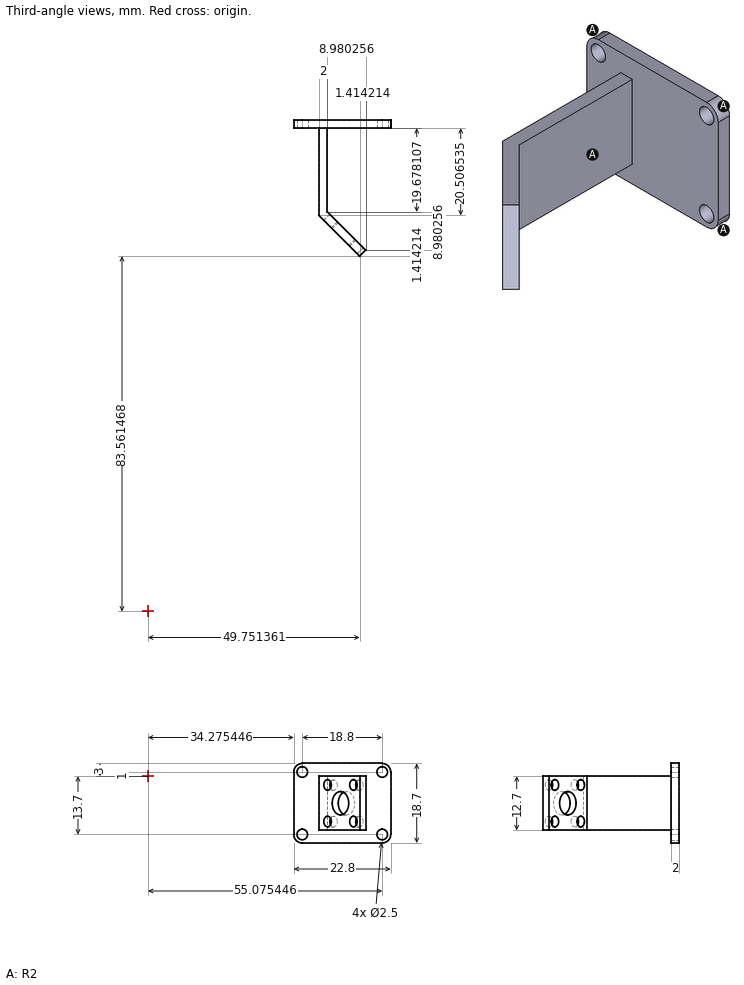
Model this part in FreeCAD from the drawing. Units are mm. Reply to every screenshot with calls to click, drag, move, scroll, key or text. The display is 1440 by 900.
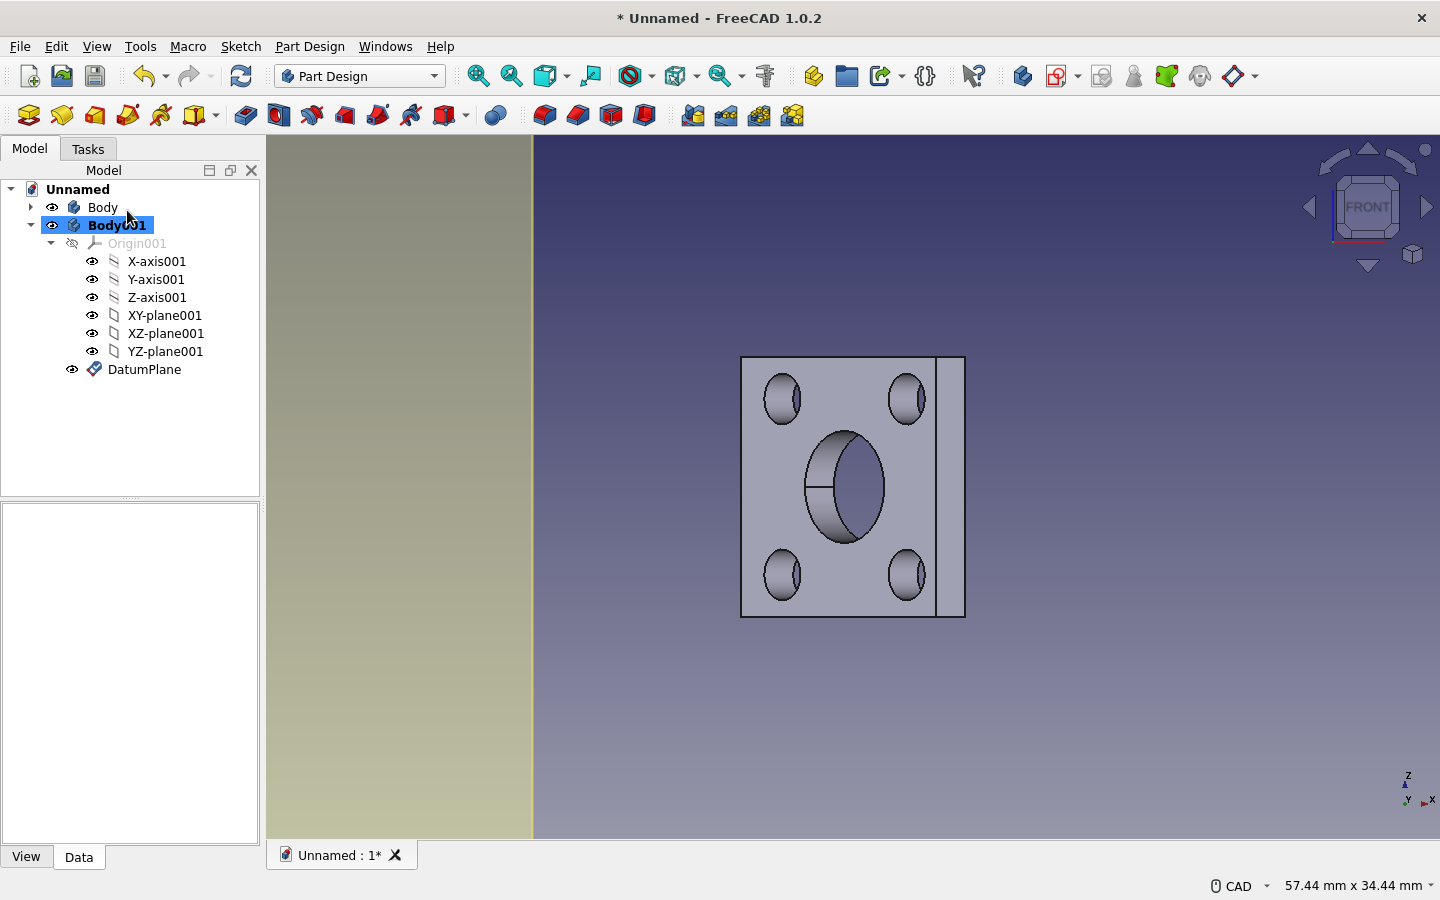
click(117, 369)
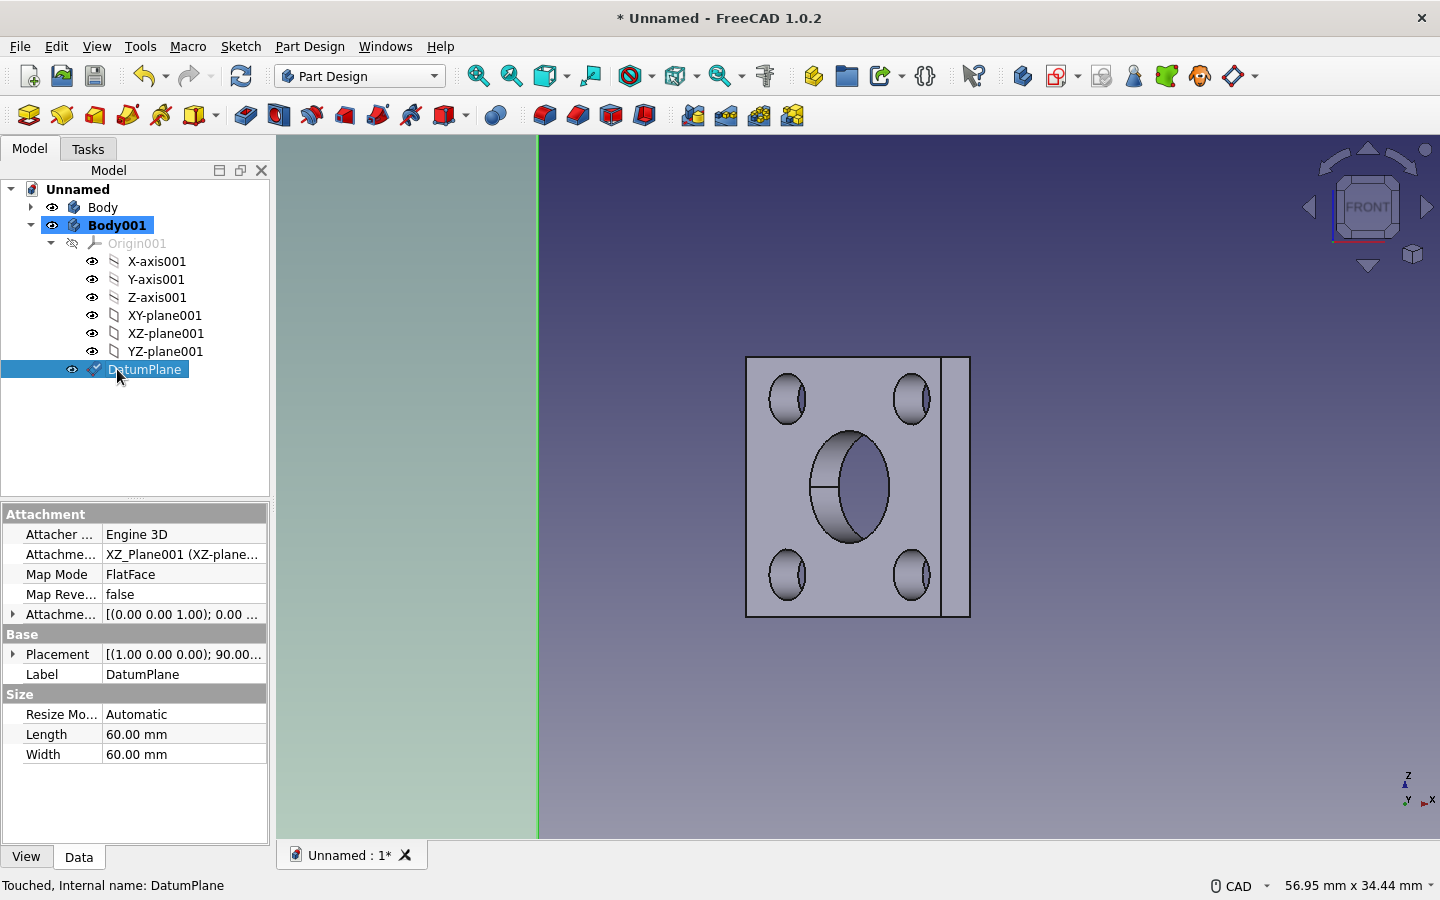
click(1056, 76)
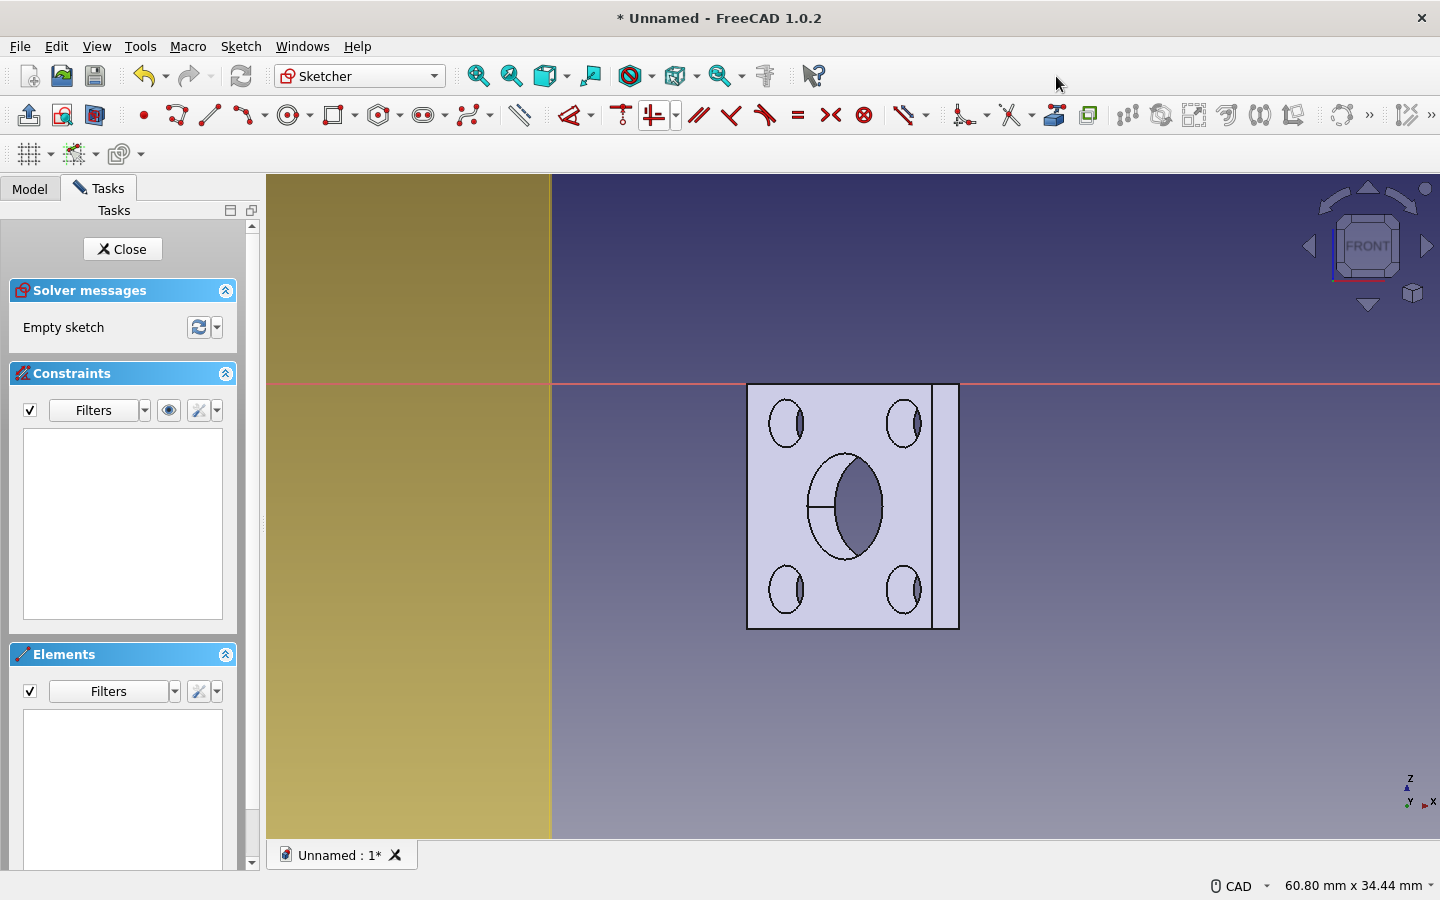
click(332, 116)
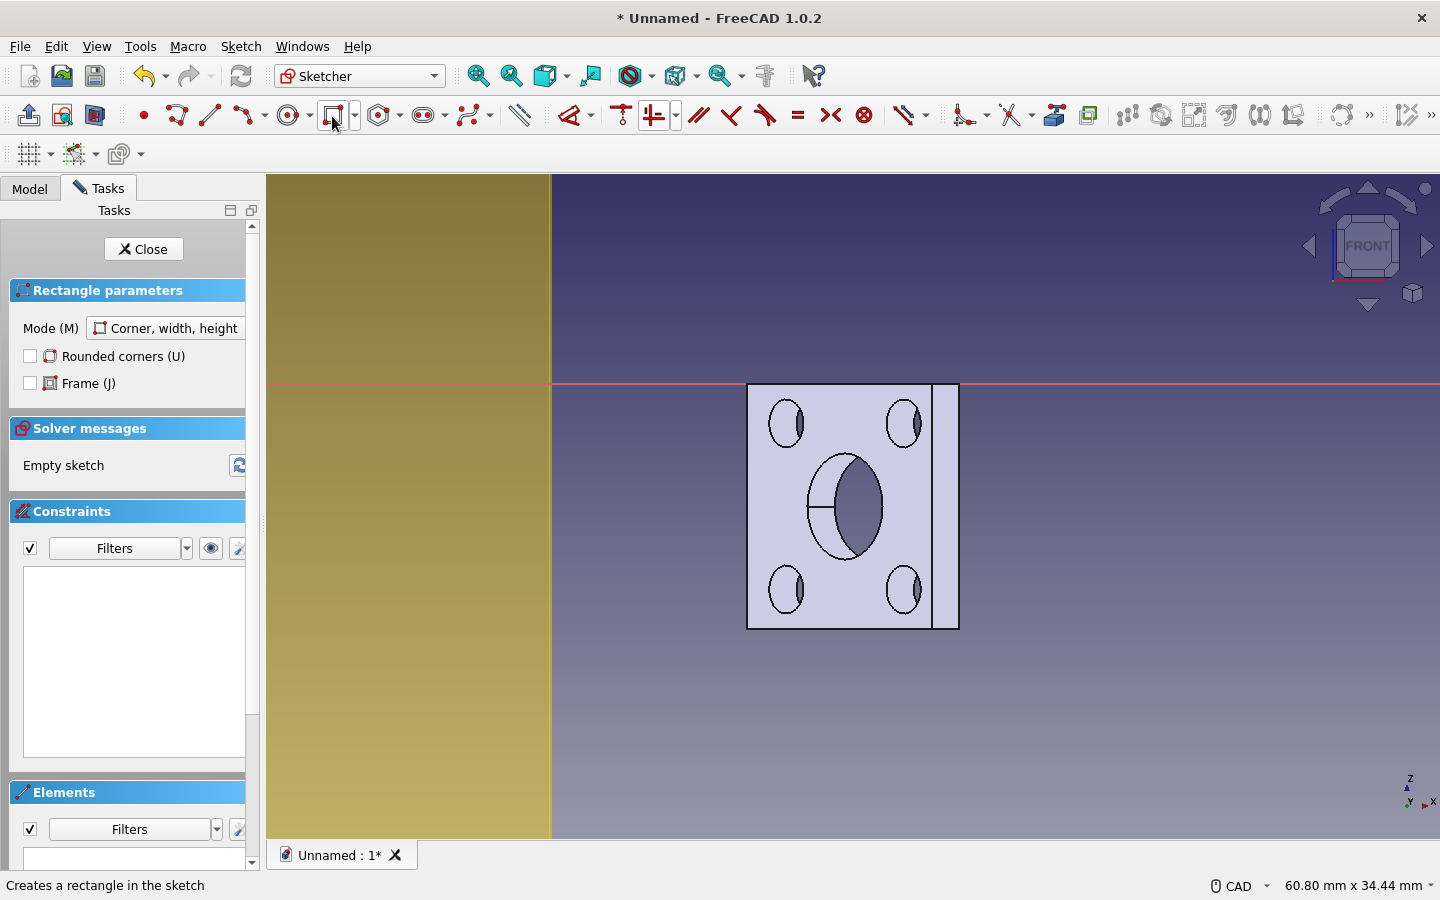
click(633, 326)
move(1073, 687)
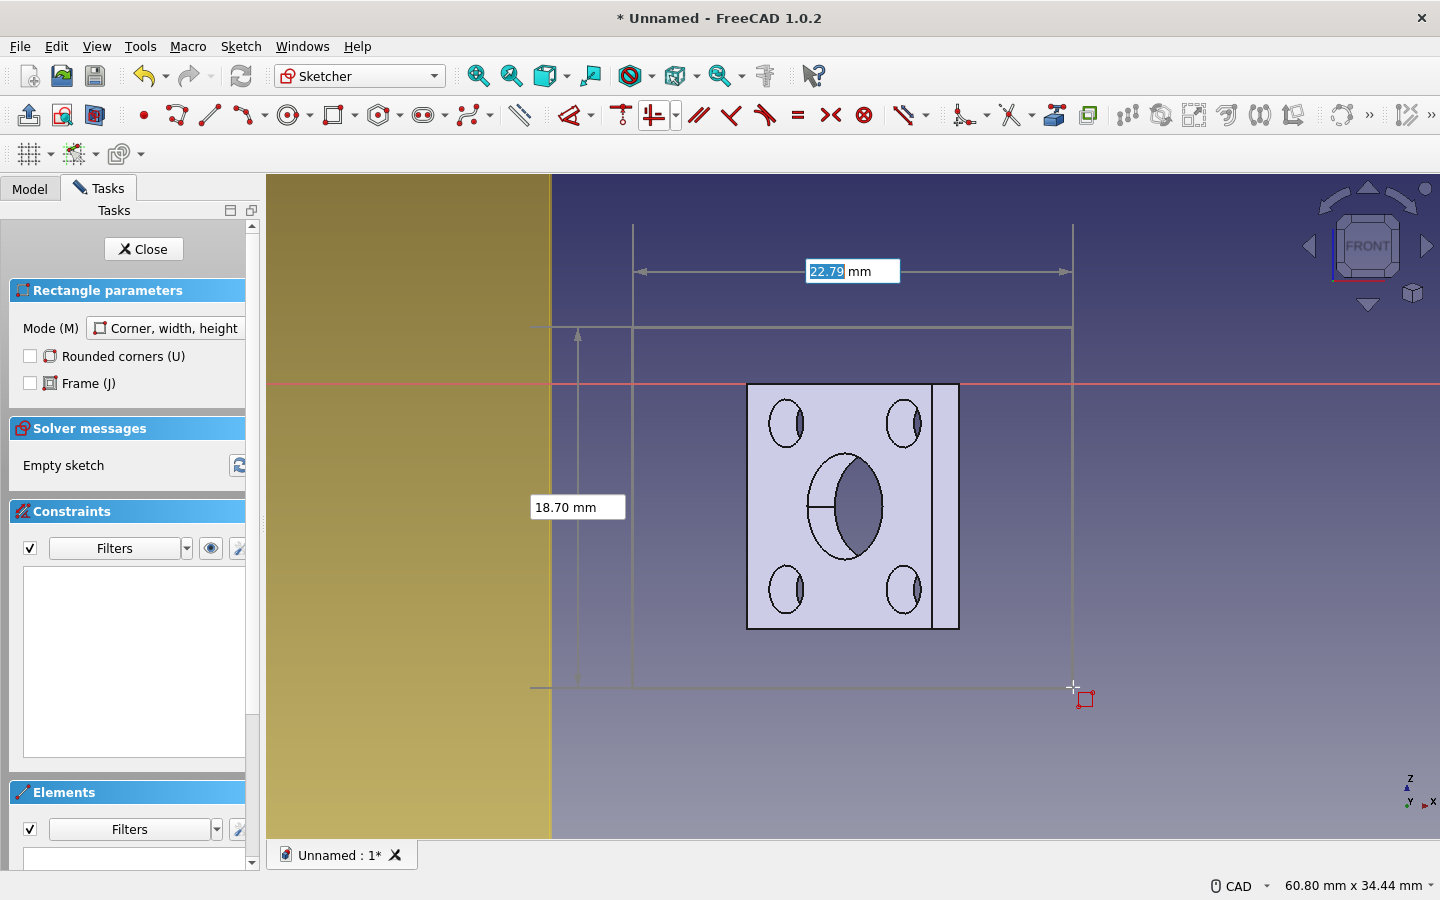
text(22.8)
key(Tab)
text(18.7)
key(Return)
key(Escape)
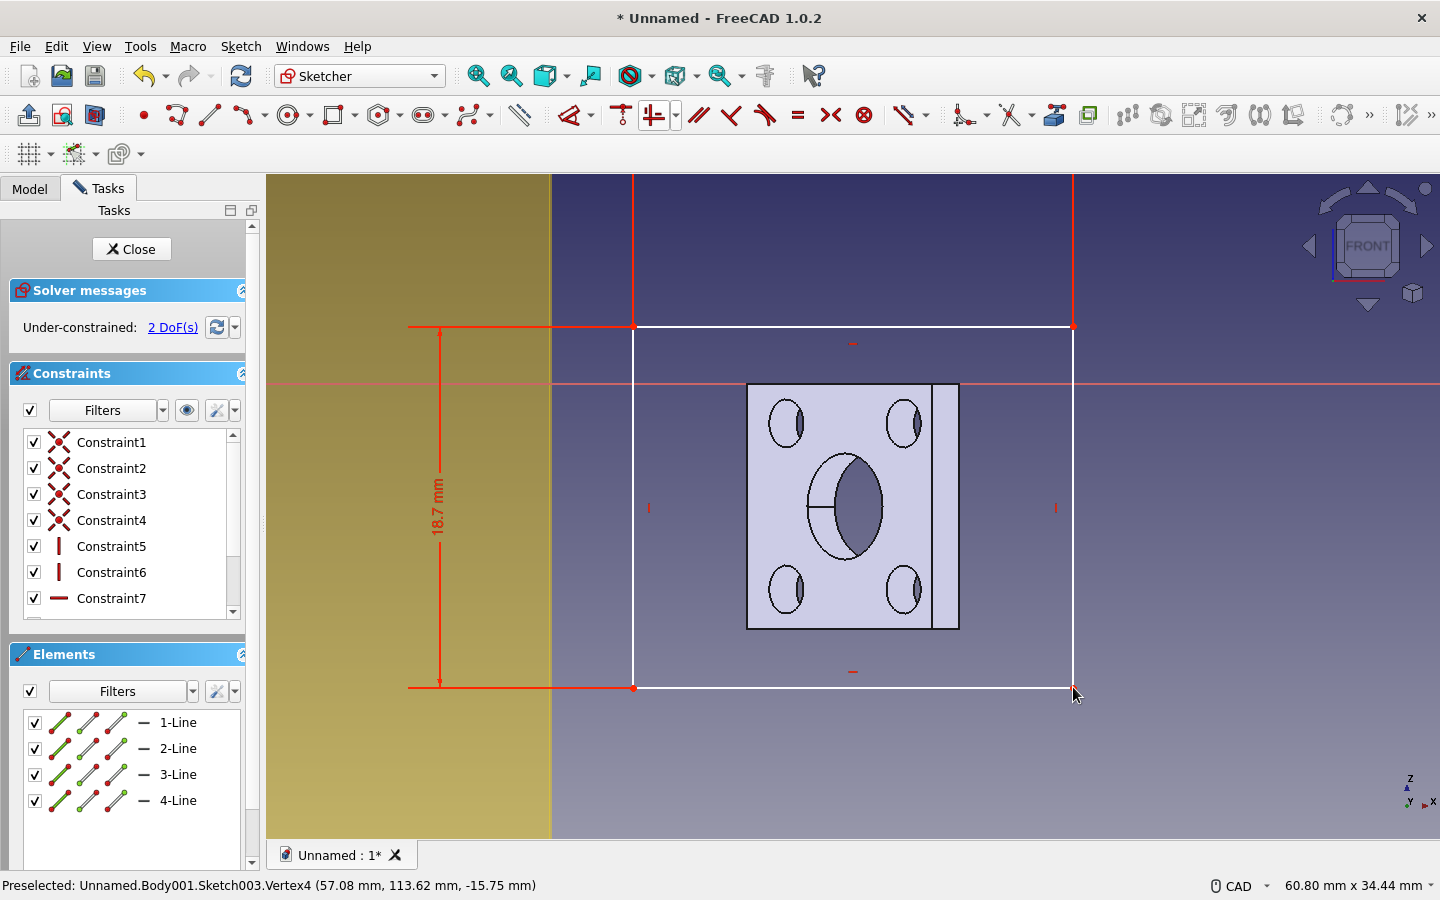
click(568, 116)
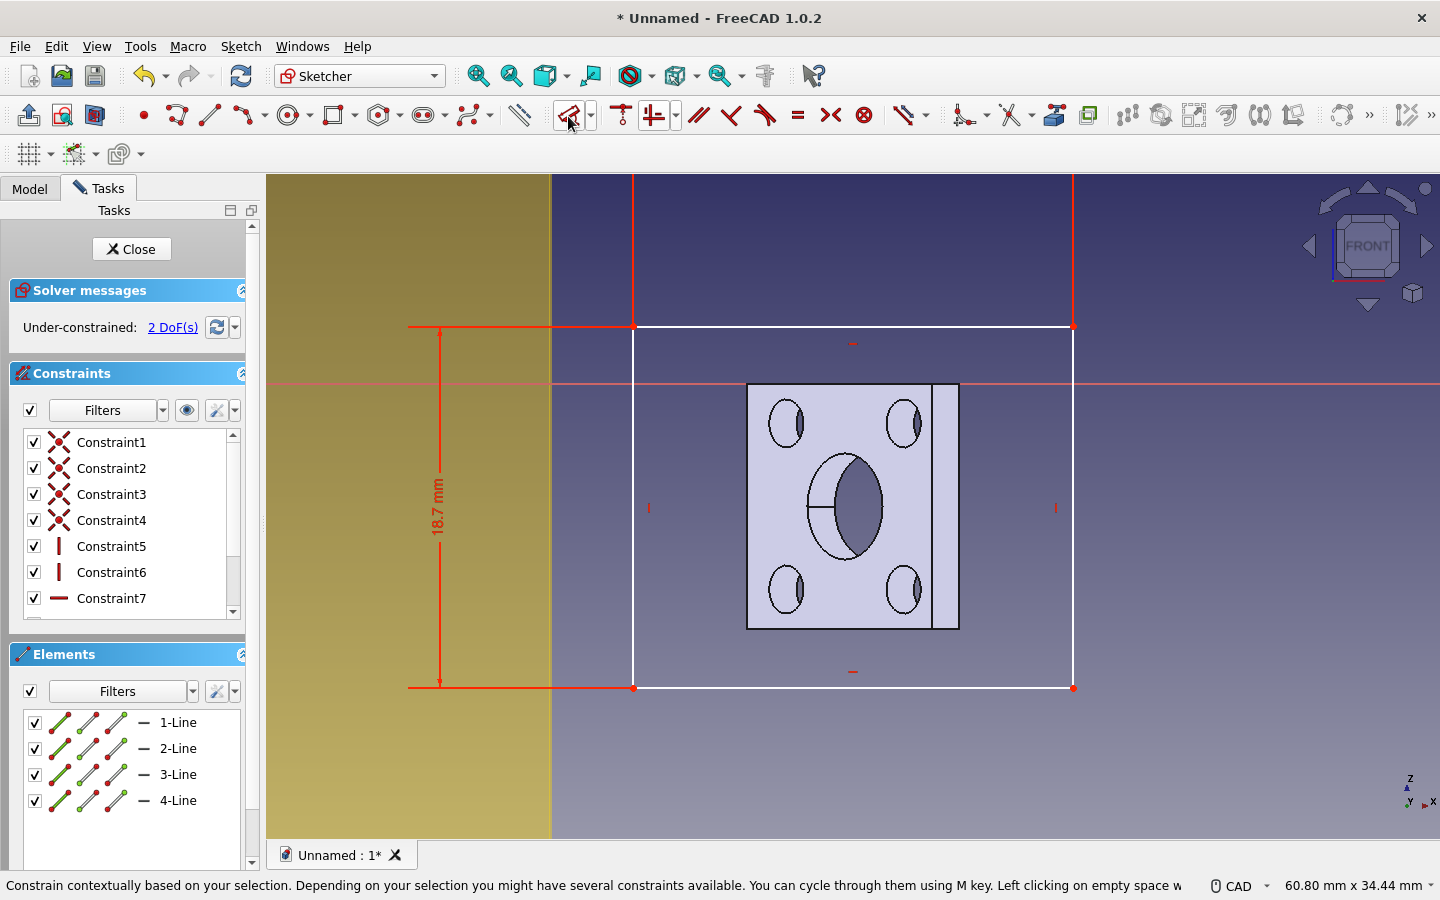
click(633, 327)
click(667, 355)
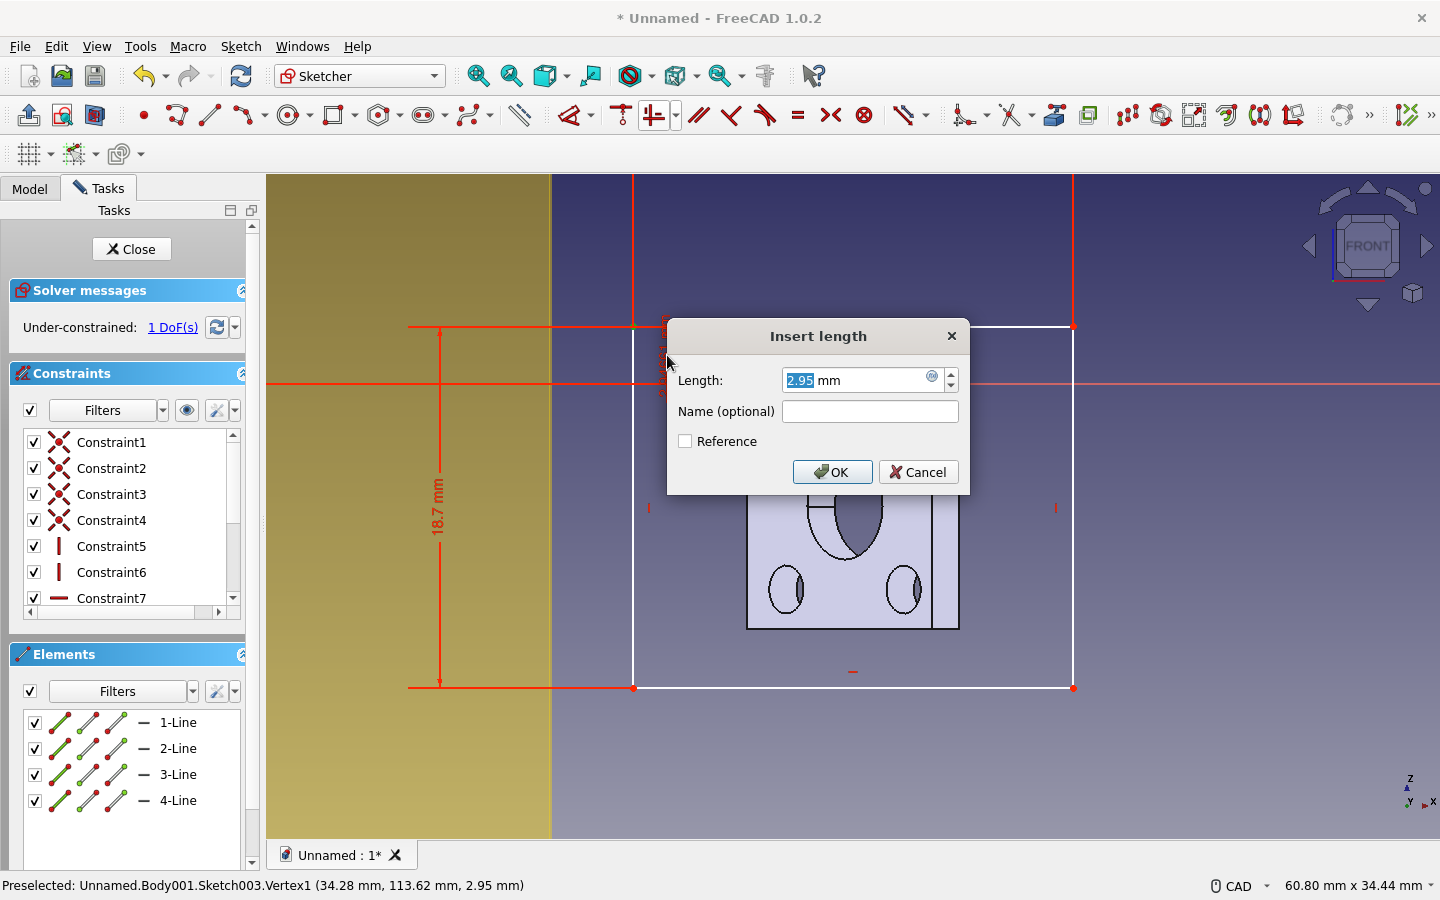
text(3)
key(Return)